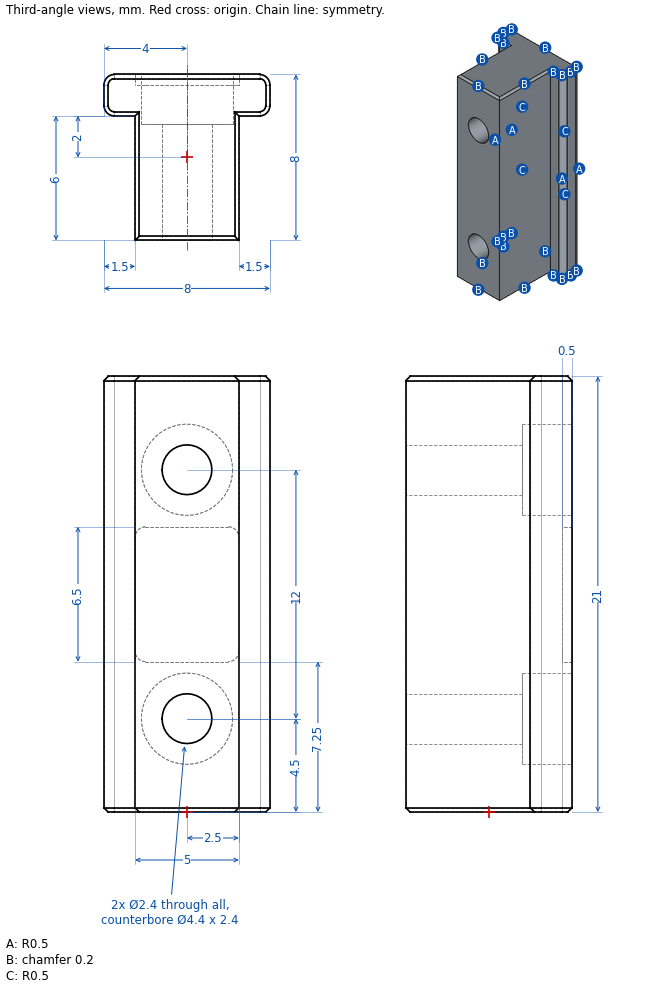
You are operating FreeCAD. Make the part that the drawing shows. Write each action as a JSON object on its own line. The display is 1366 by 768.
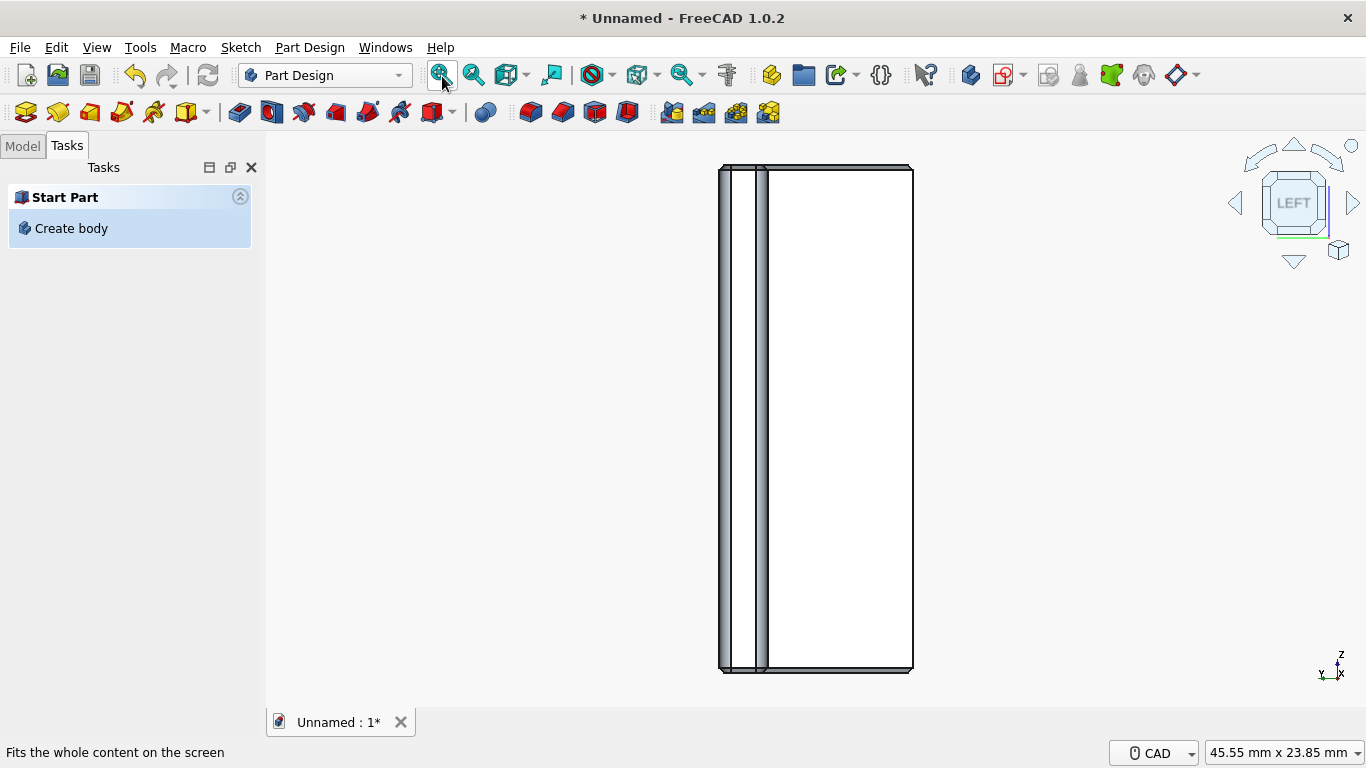
{"action": "key", "text": "v 3"}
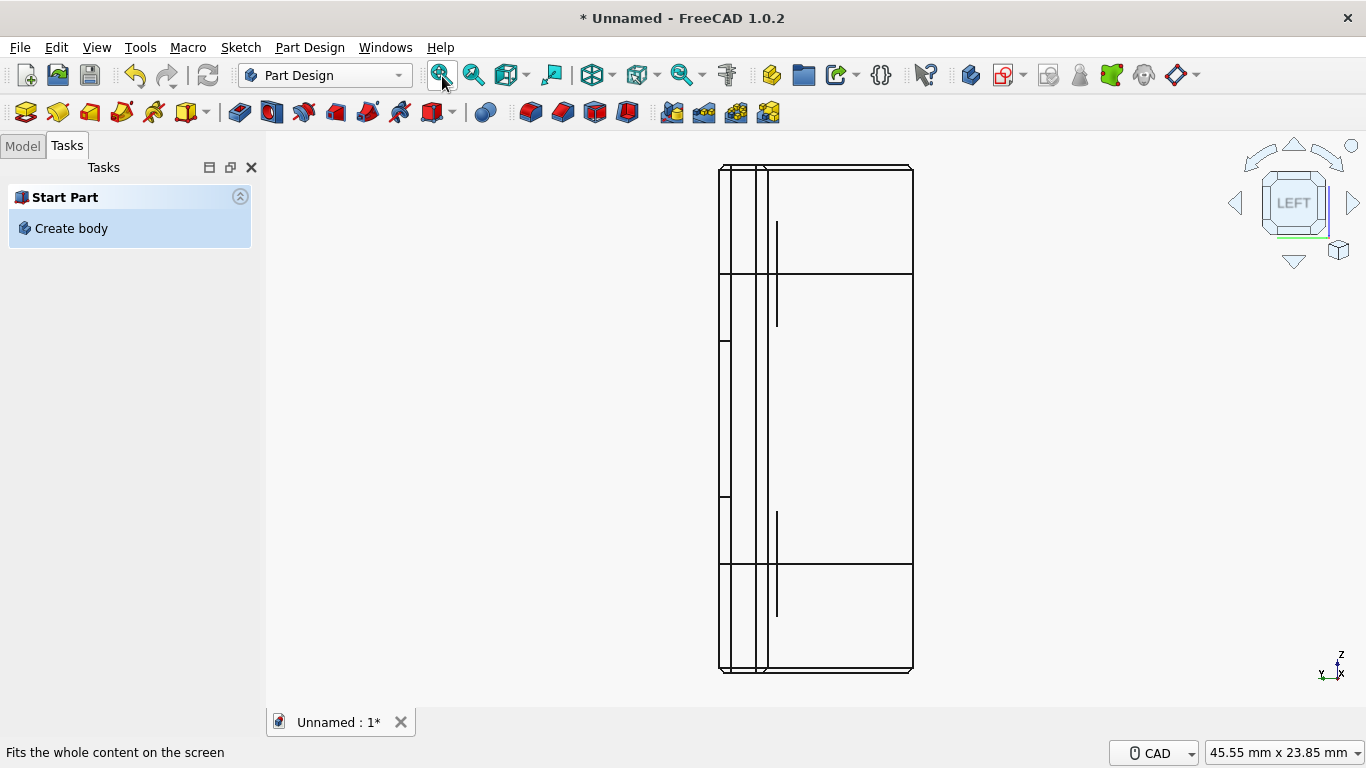
{"action": "key", "text": "0"}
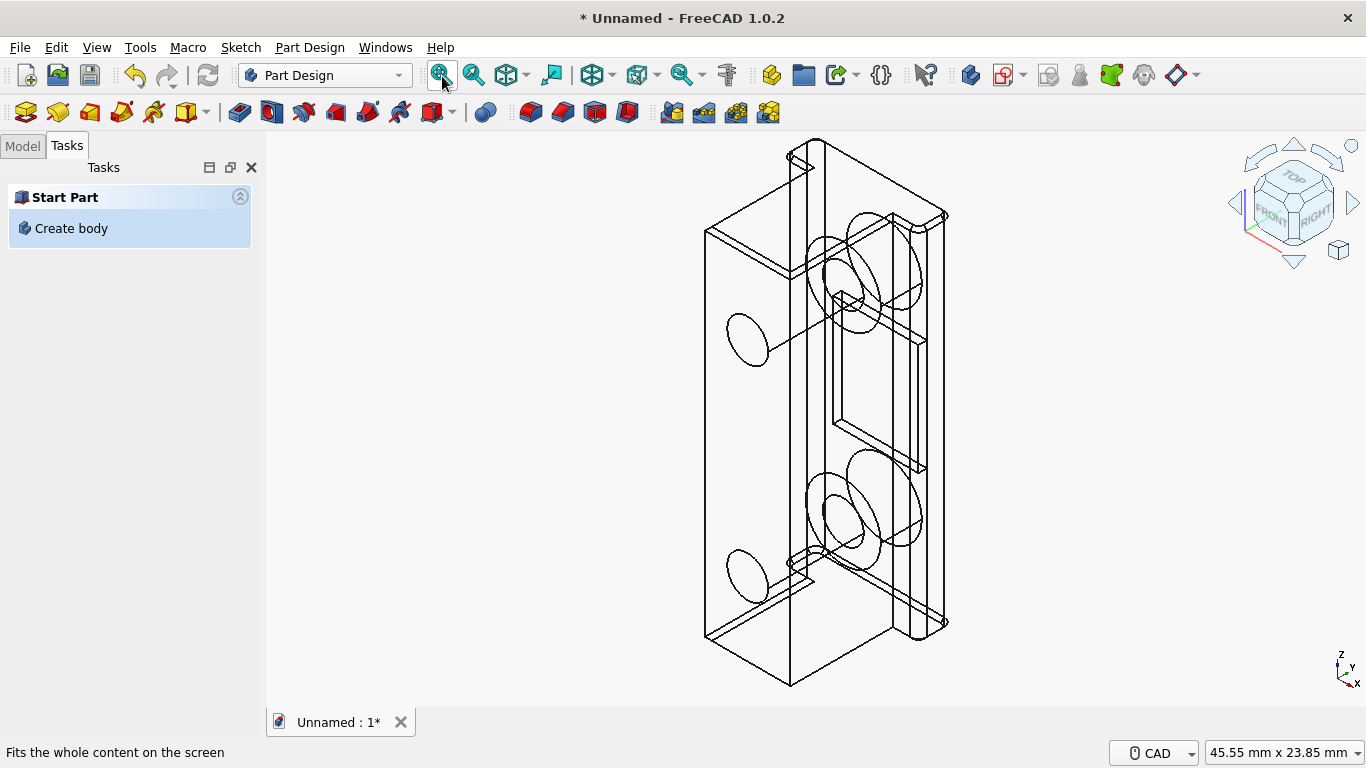
{"action": "scroll", "coordinate": [923, 470], "scroll_direction": "up", "scroll_amount": 6}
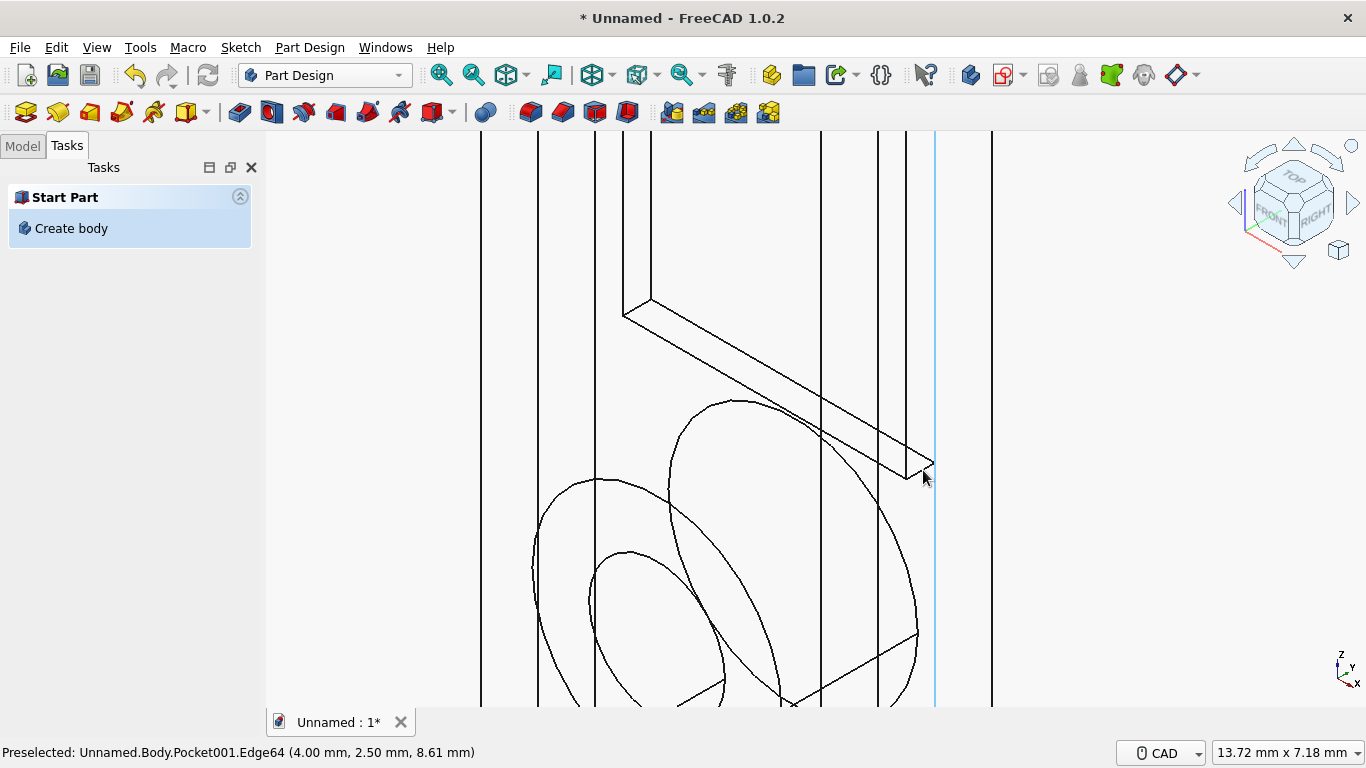
{"action": "left_click", "coordinate": [921, 470]}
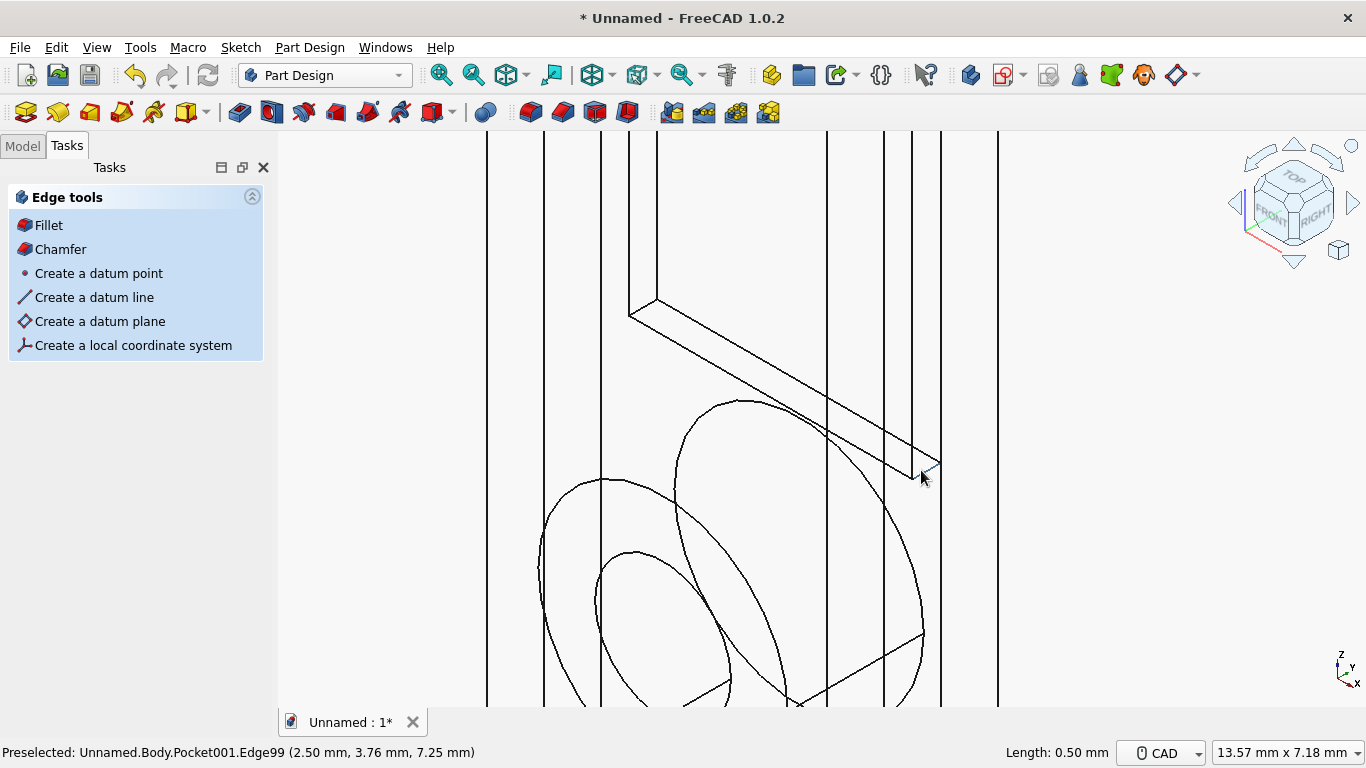
{"action": "left_click", "coordinate": [643, 306], "text": "ctrl"}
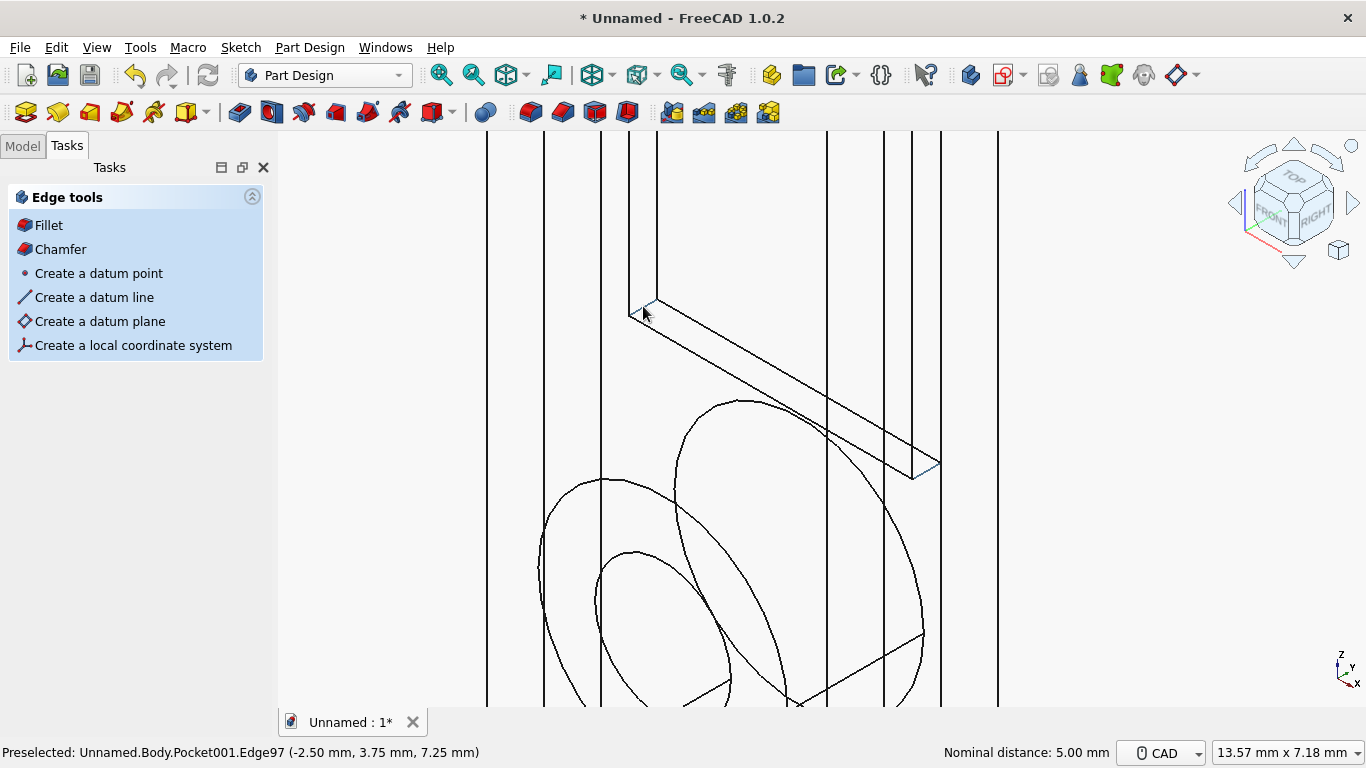
{"action": "left_click", "coordinate": [442, 76]}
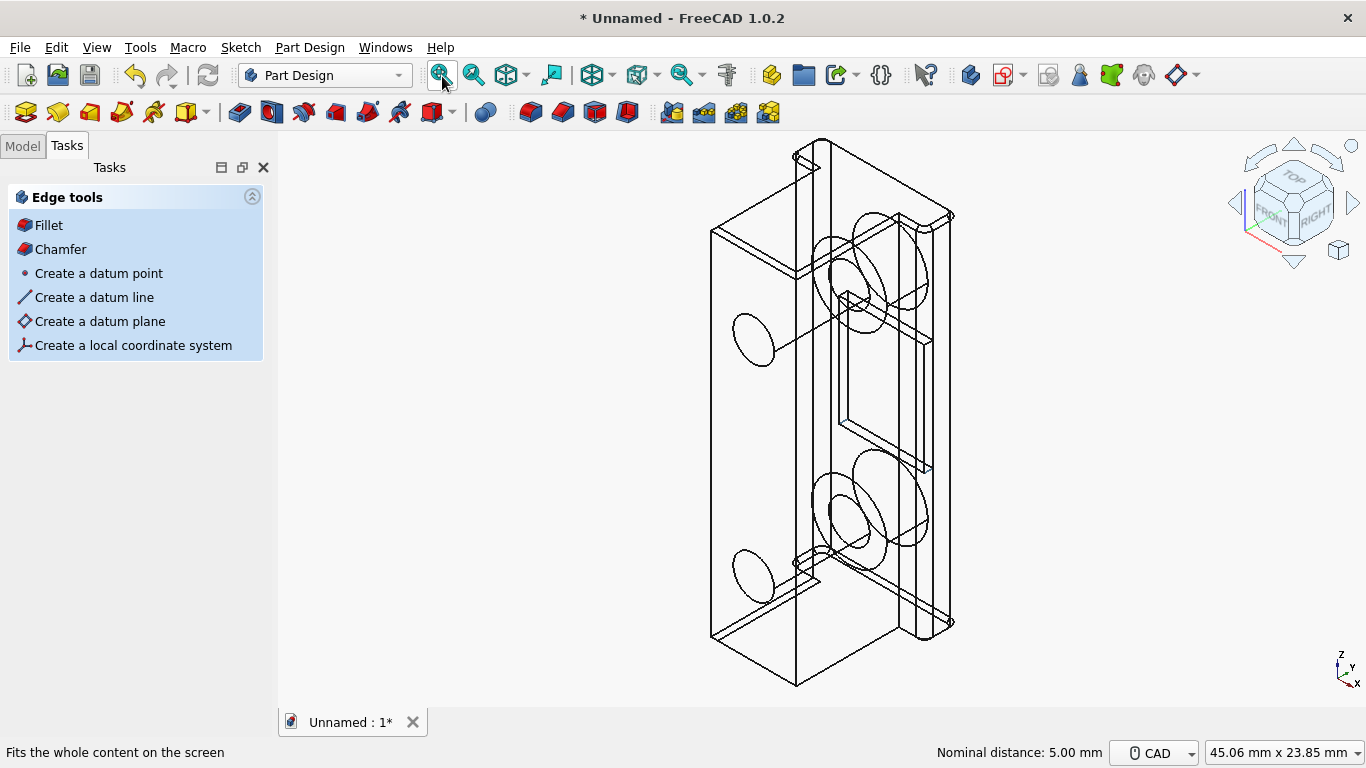
{"action": "key", "text": "2"}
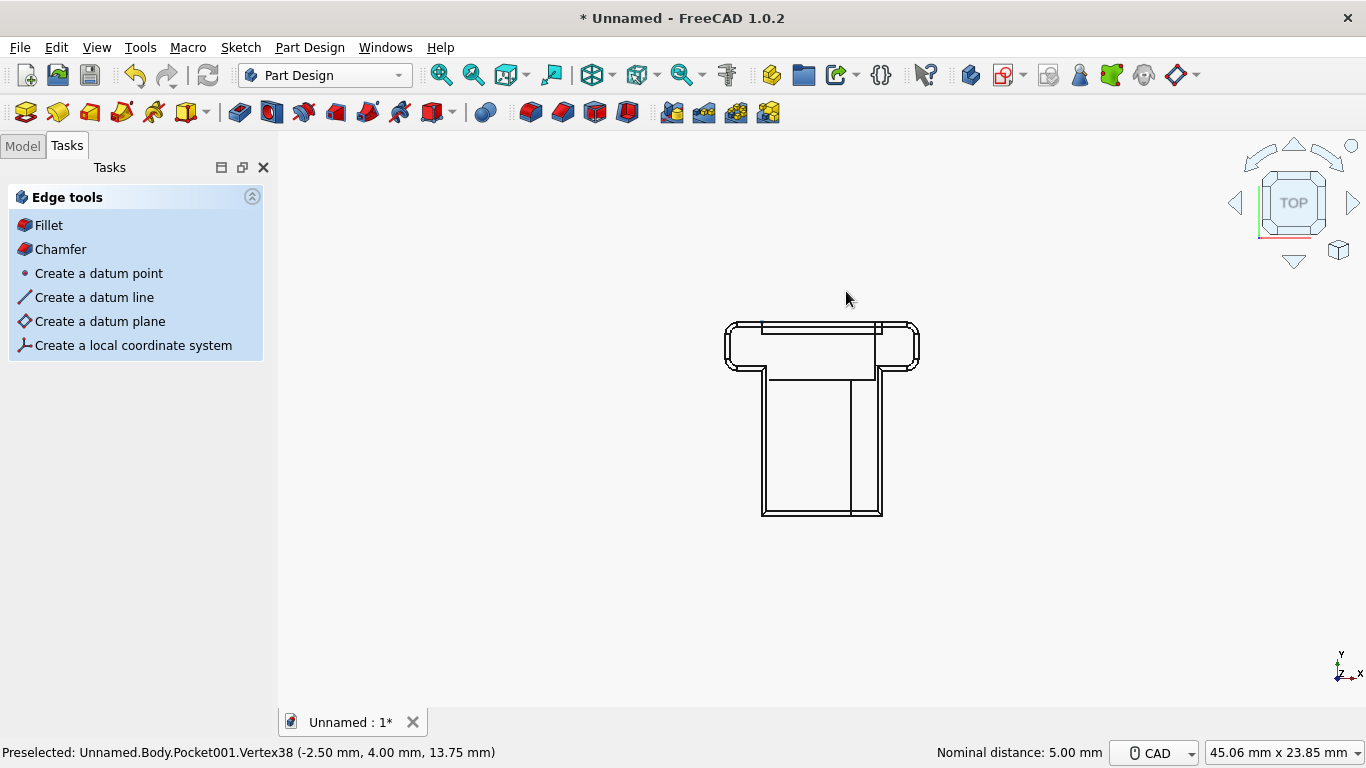
{"action": "left_click", "coordinate": [442, 76]}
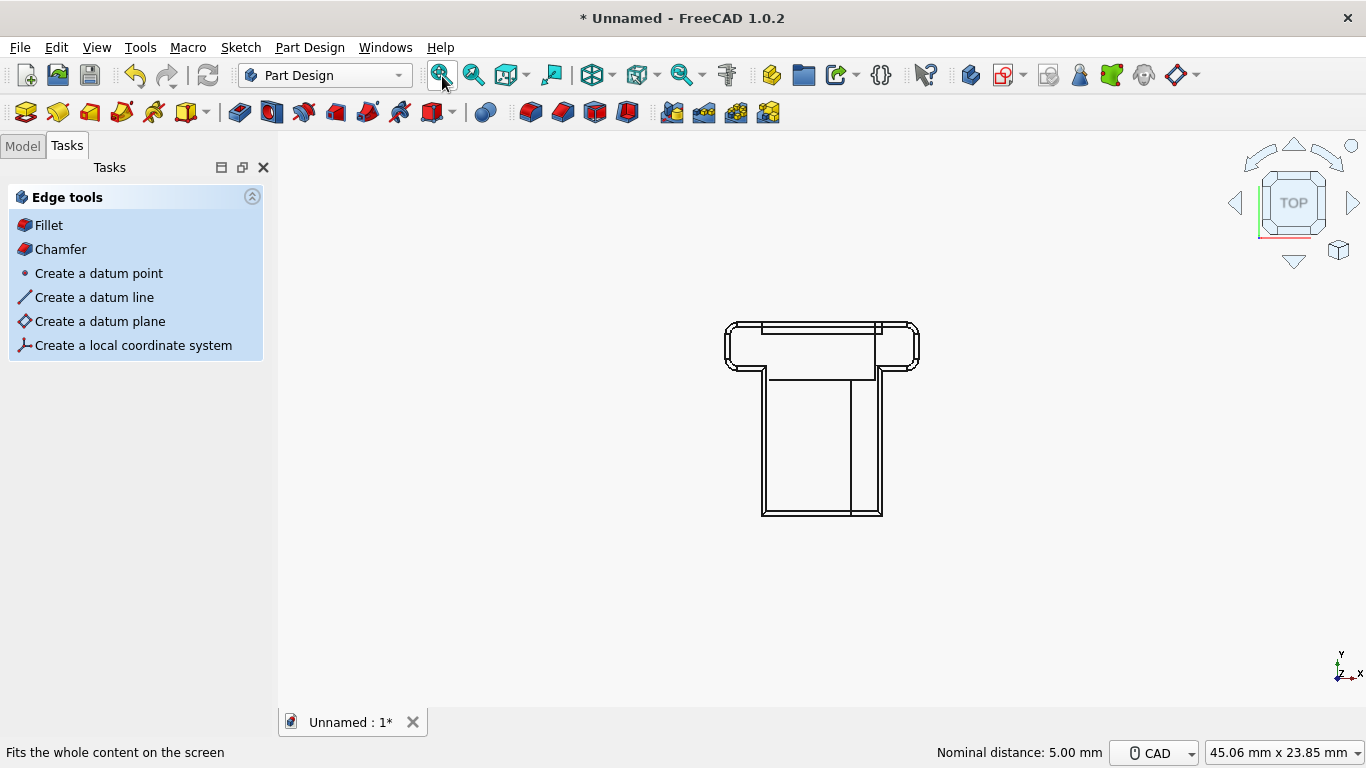
{"action": "scroll", "coordinate": [882, 327], "scroll_direction": "up", "scroll_amount": 6}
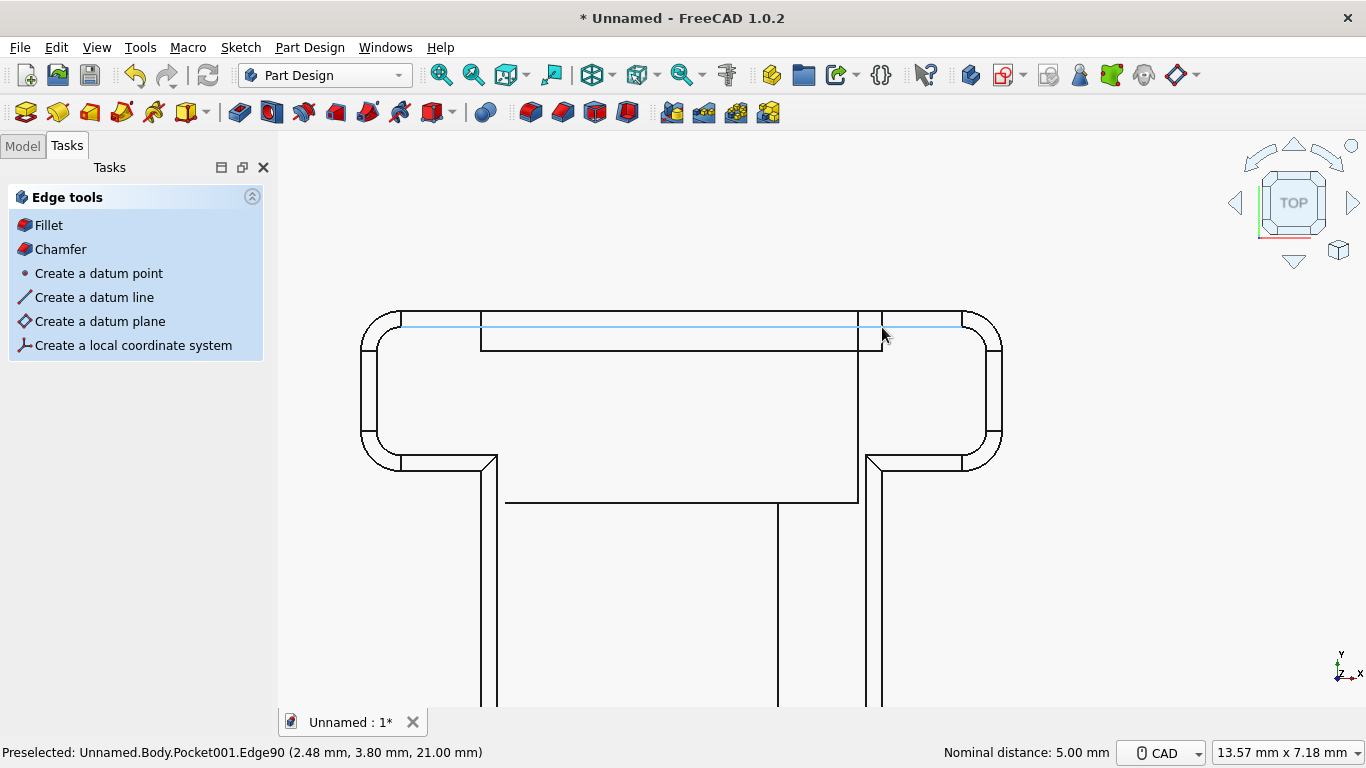
{"action": "left_click", "coordinate": [882, 334], "text": "ctrl"}